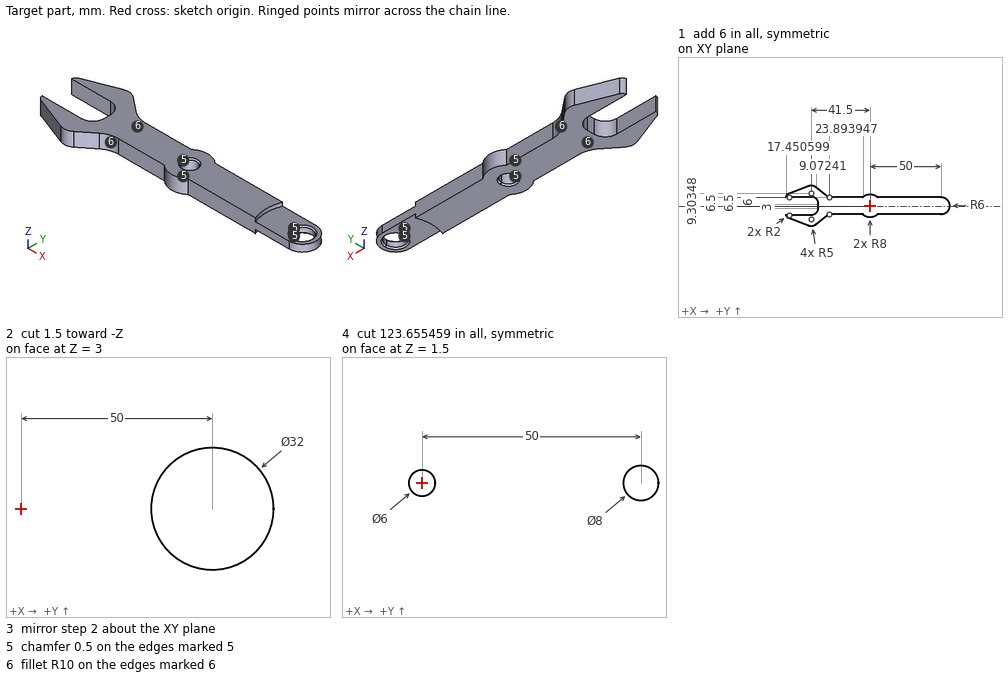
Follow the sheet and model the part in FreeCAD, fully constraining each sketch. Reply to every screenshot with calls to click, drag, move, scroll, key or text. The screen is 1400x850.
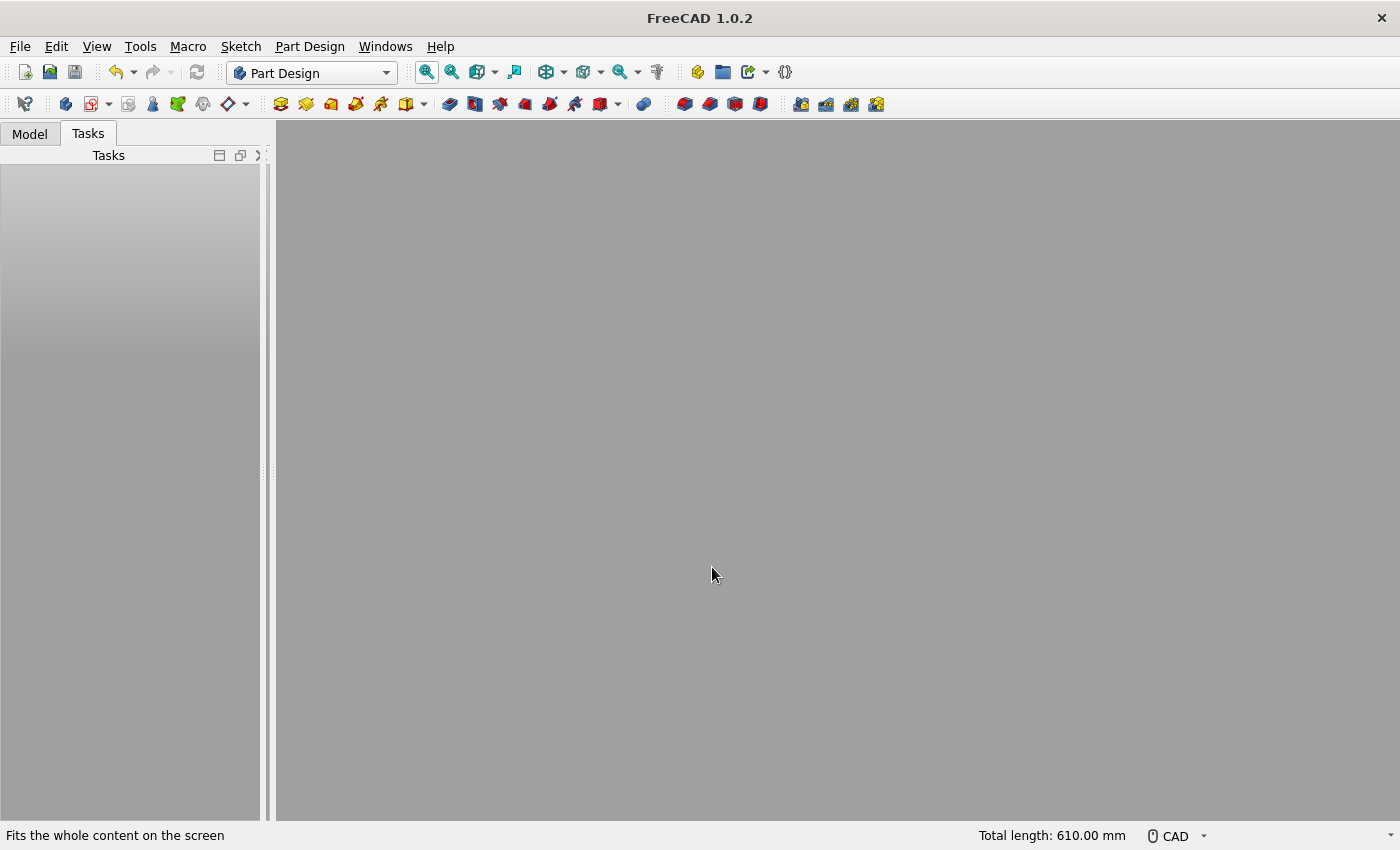
click(25, 72)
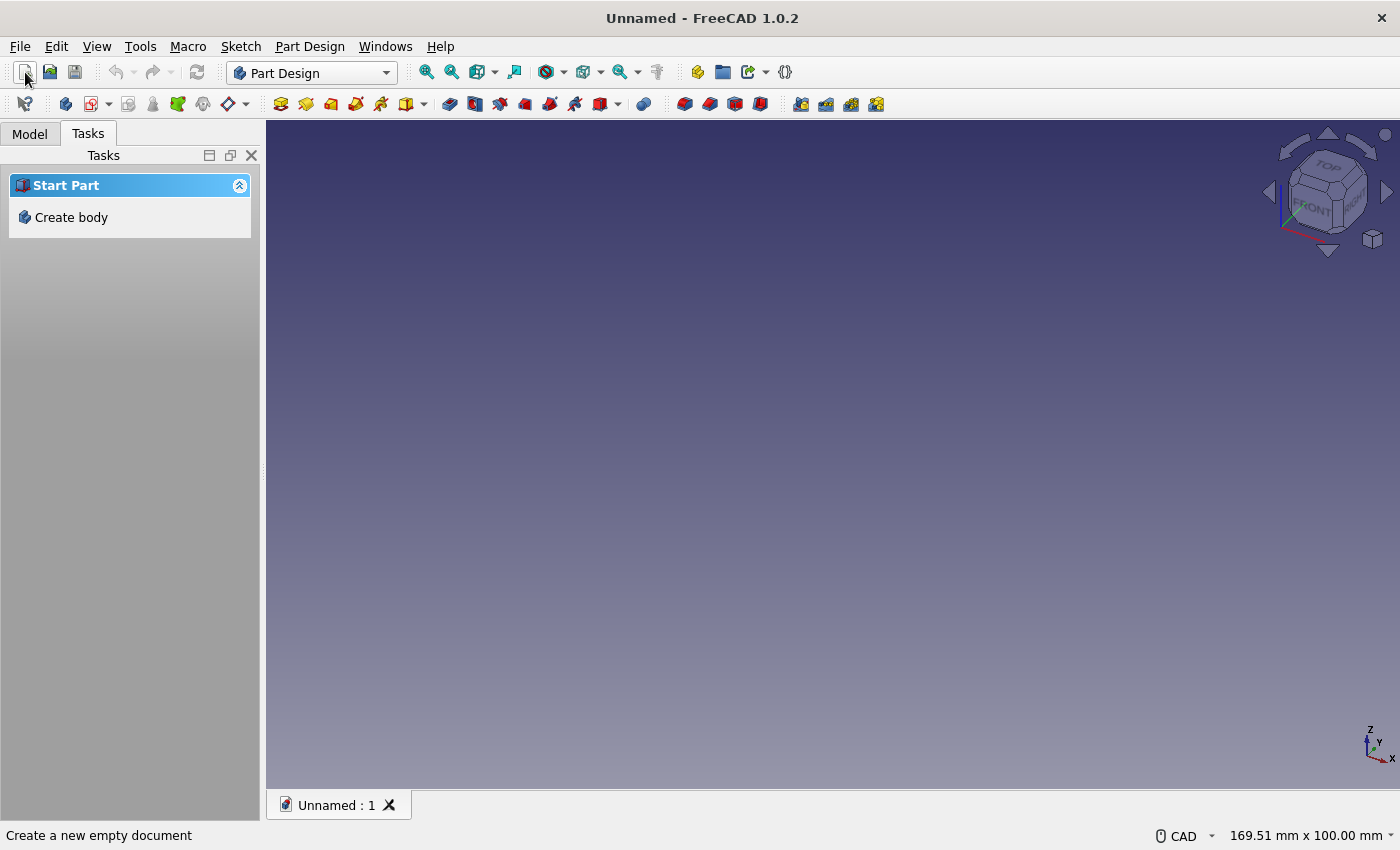
click(90, 104)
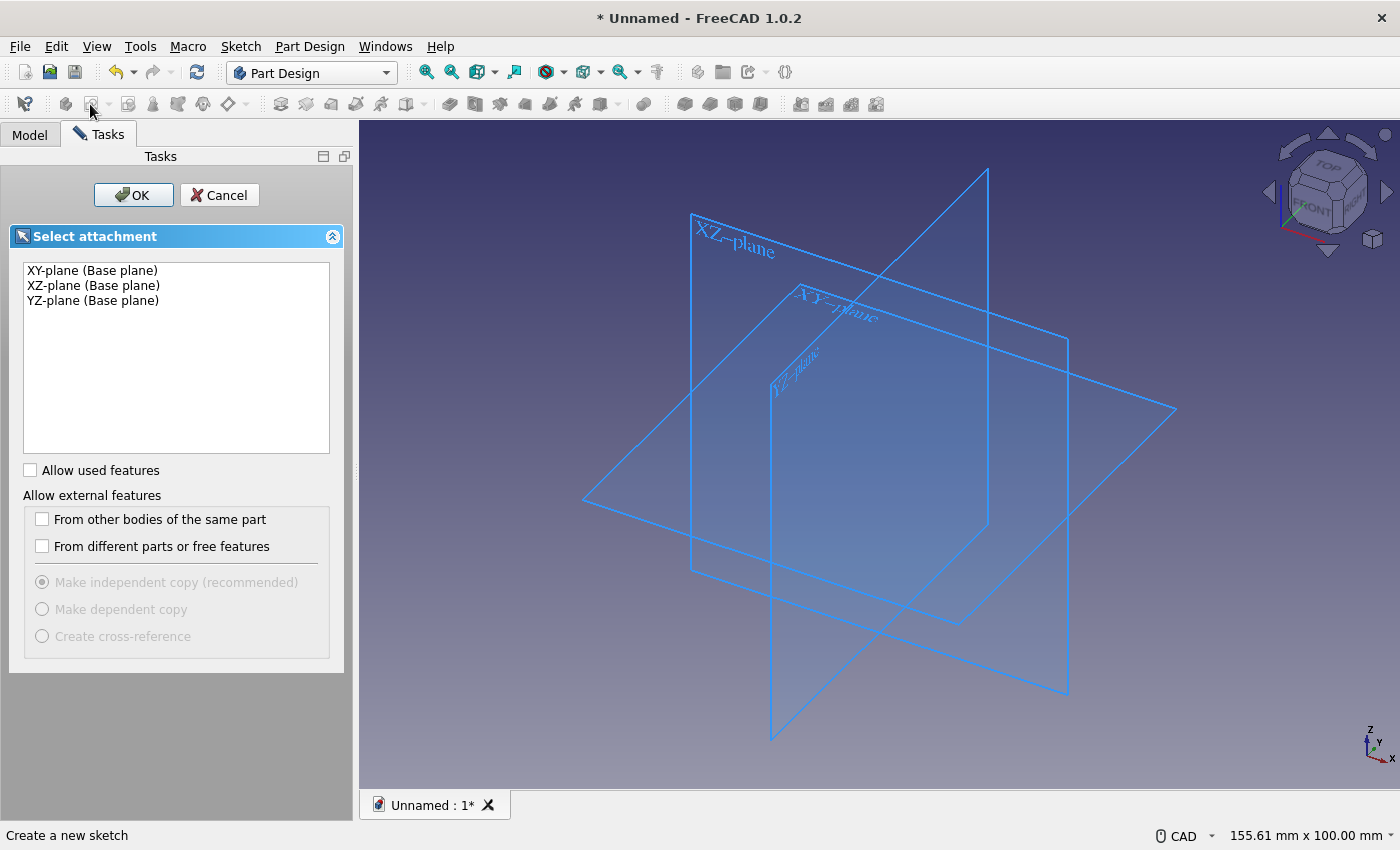
click(84, 270)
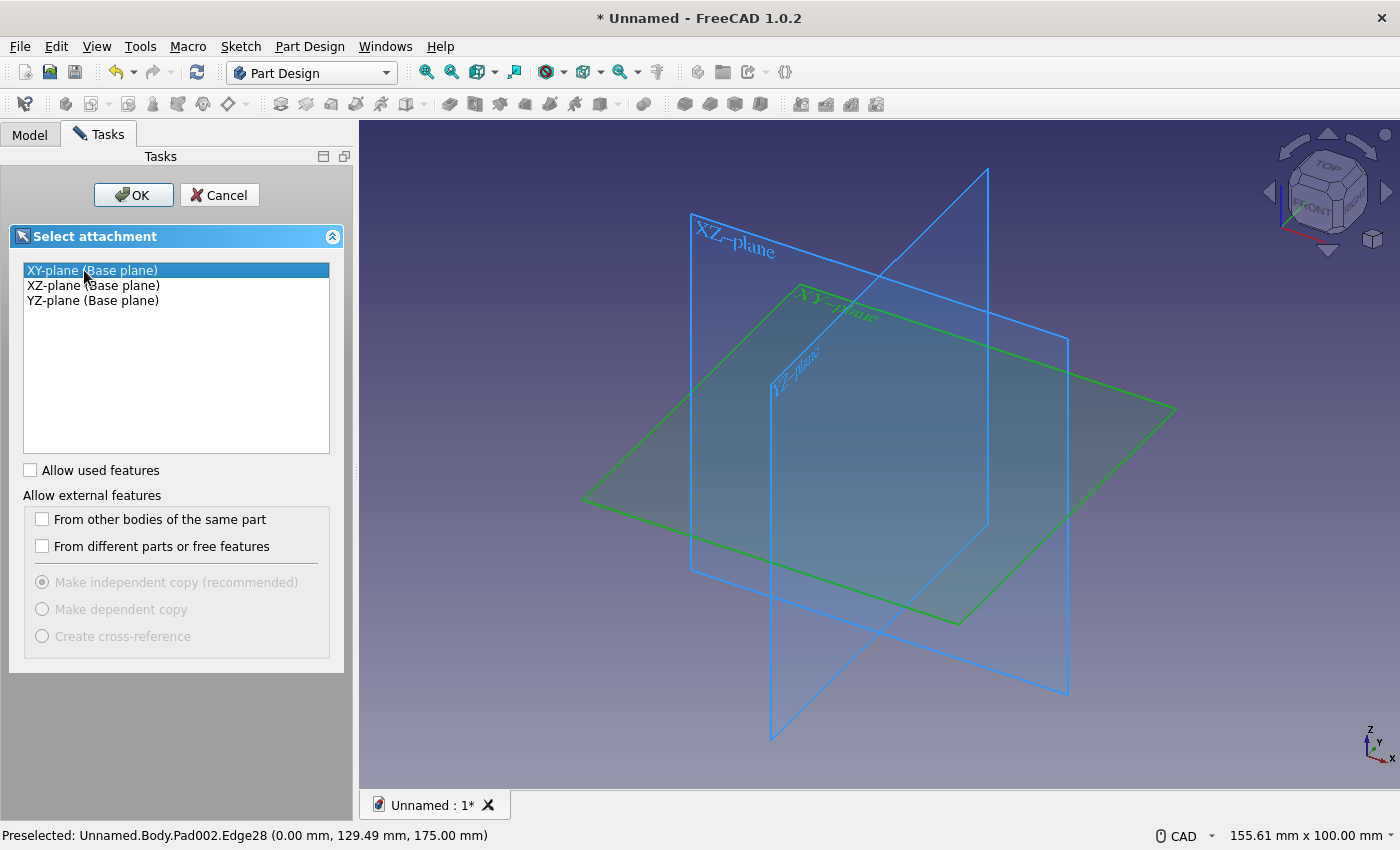
click(134, 195)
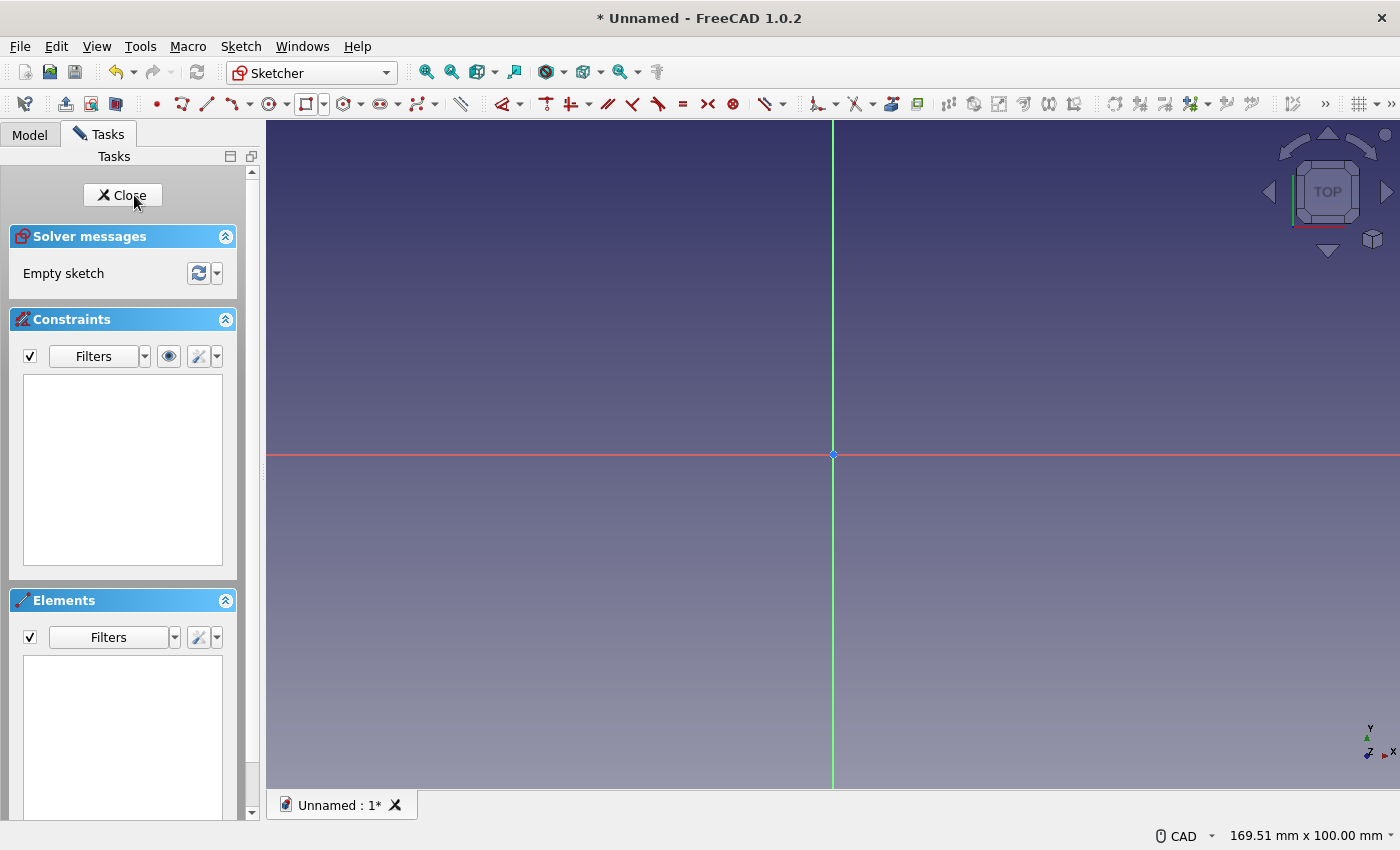
click(207, 104)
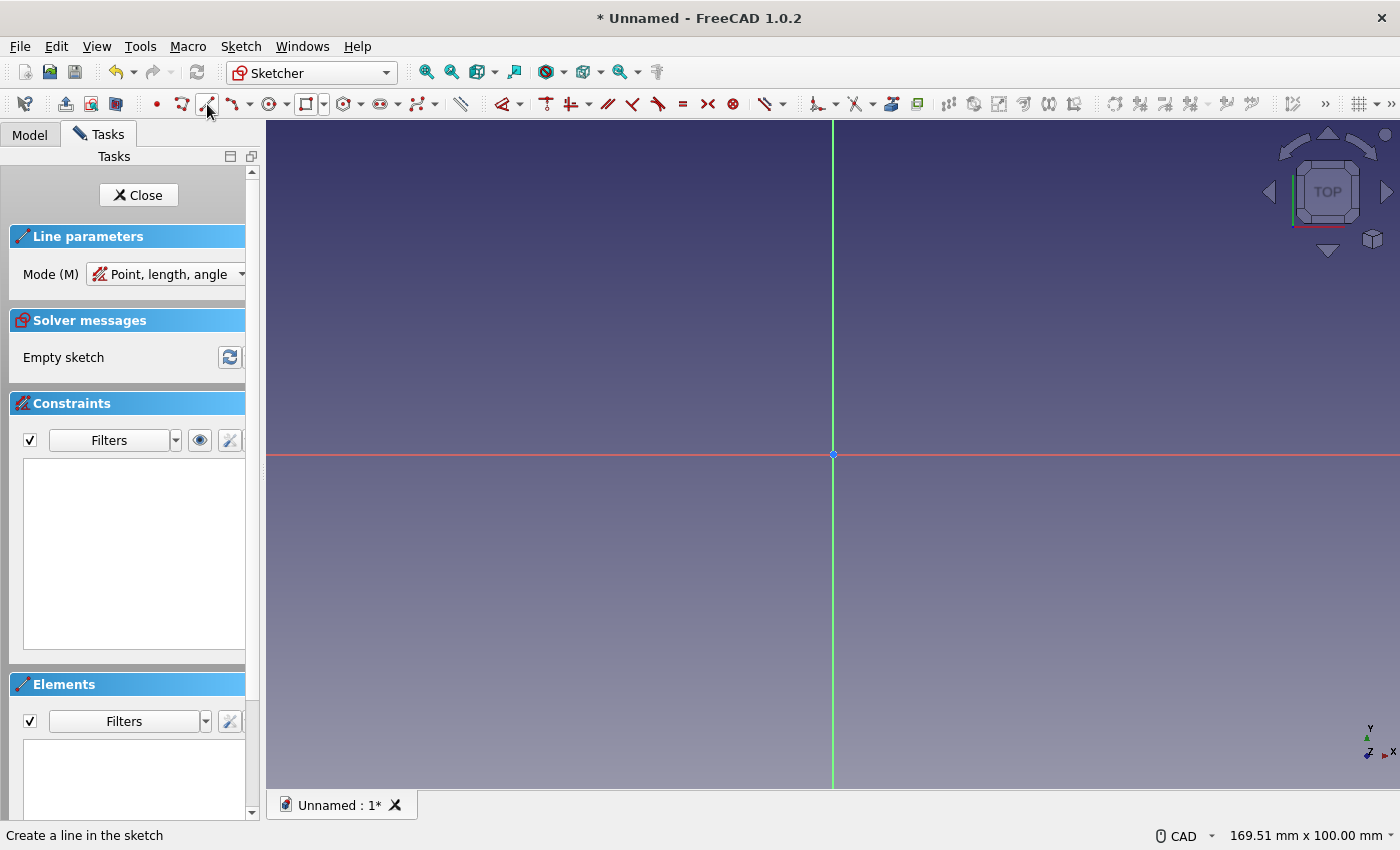
click(1168, 414)
click(868, 414)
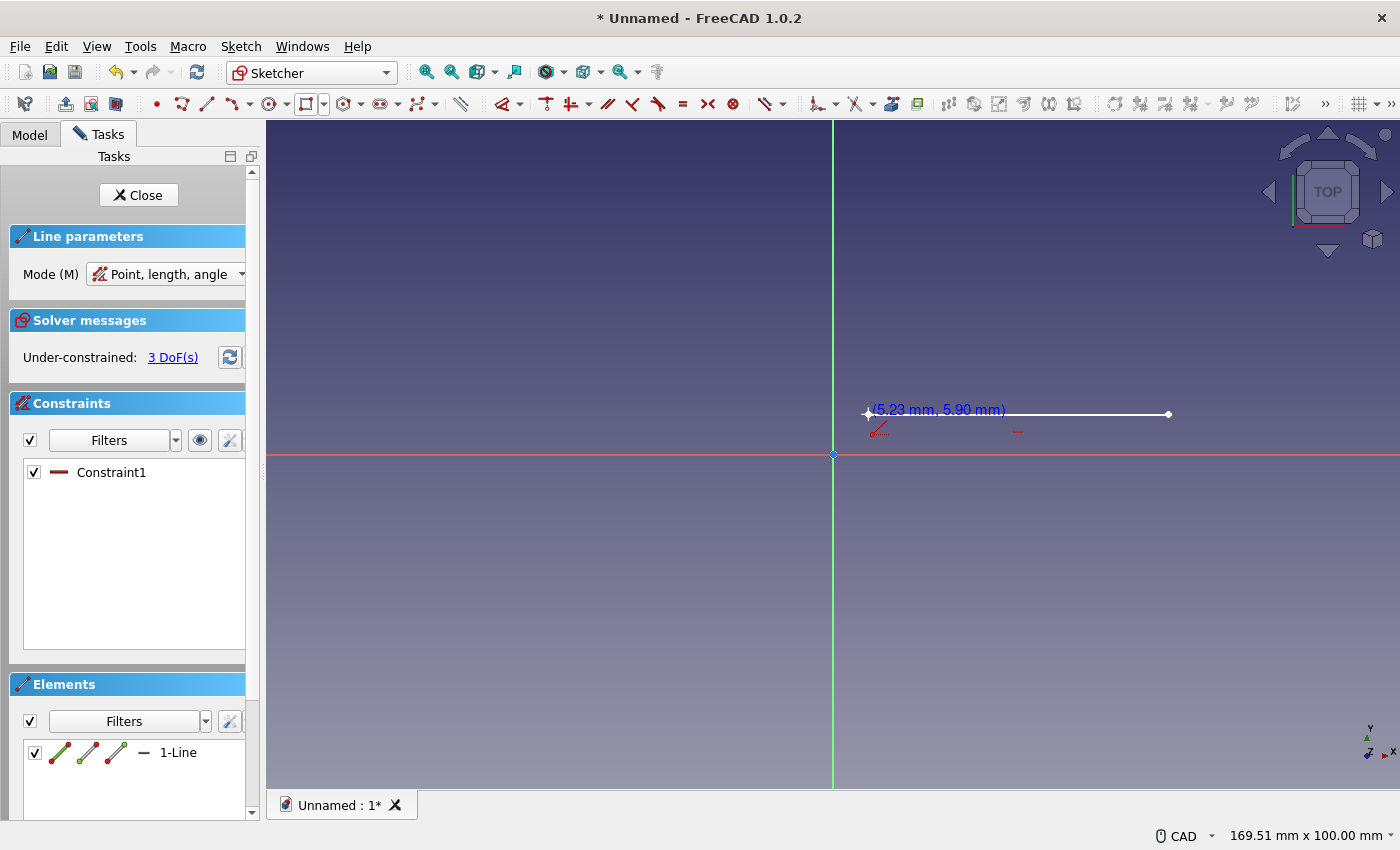
click(182, 104)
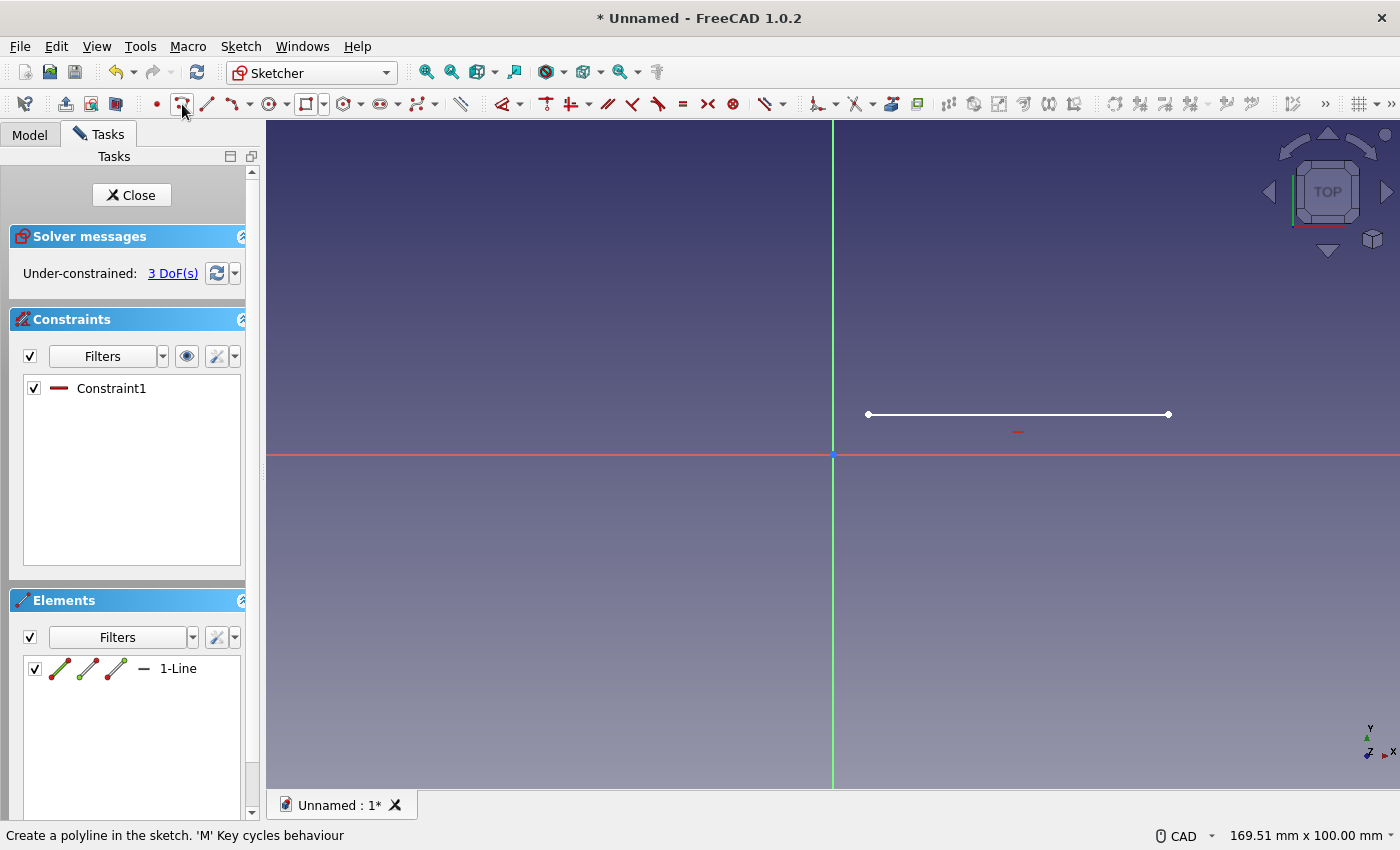
click(798, 414)
click(638, 414)
click(577, 366)
right_click(577, 366)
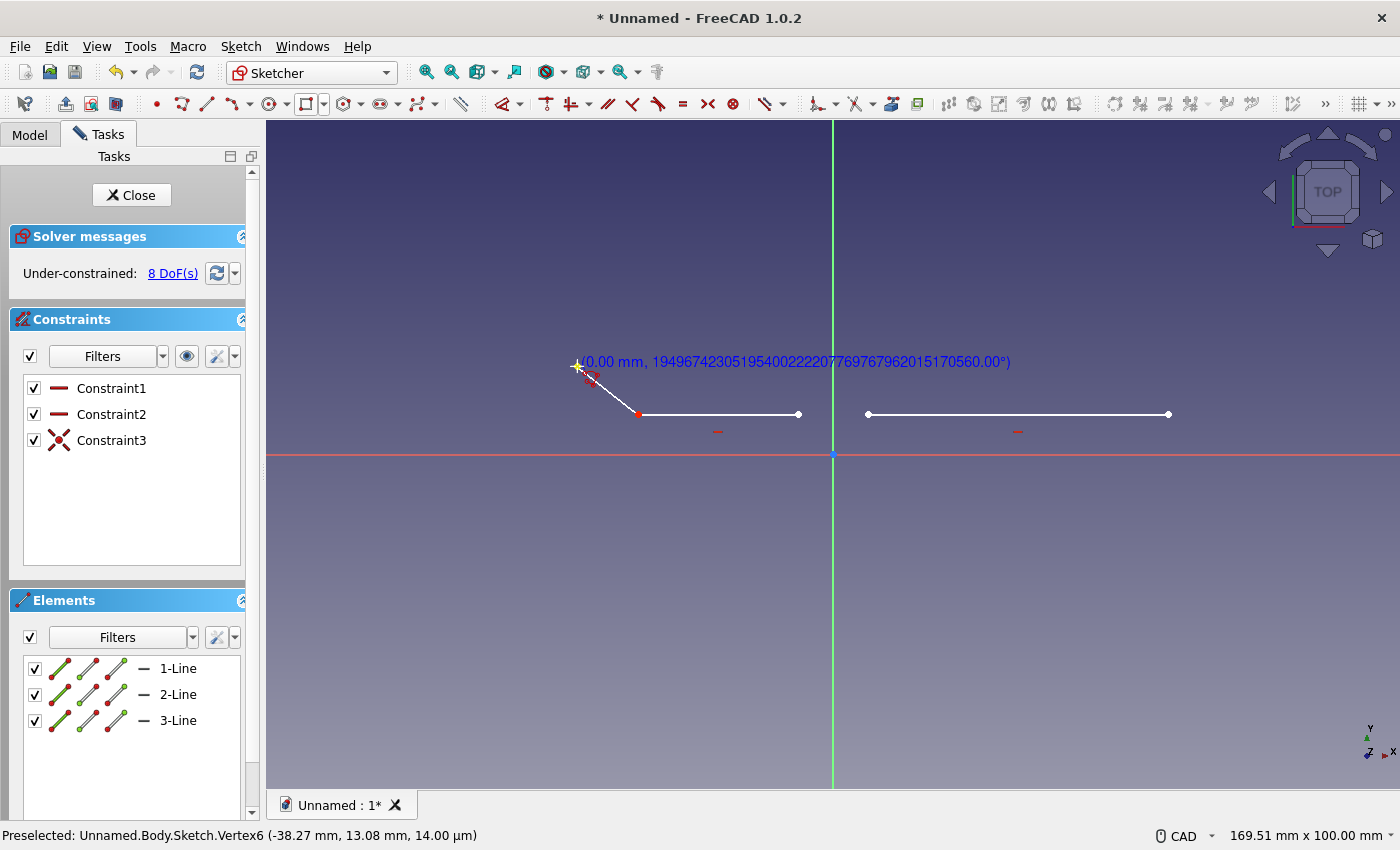
click(207, 104)